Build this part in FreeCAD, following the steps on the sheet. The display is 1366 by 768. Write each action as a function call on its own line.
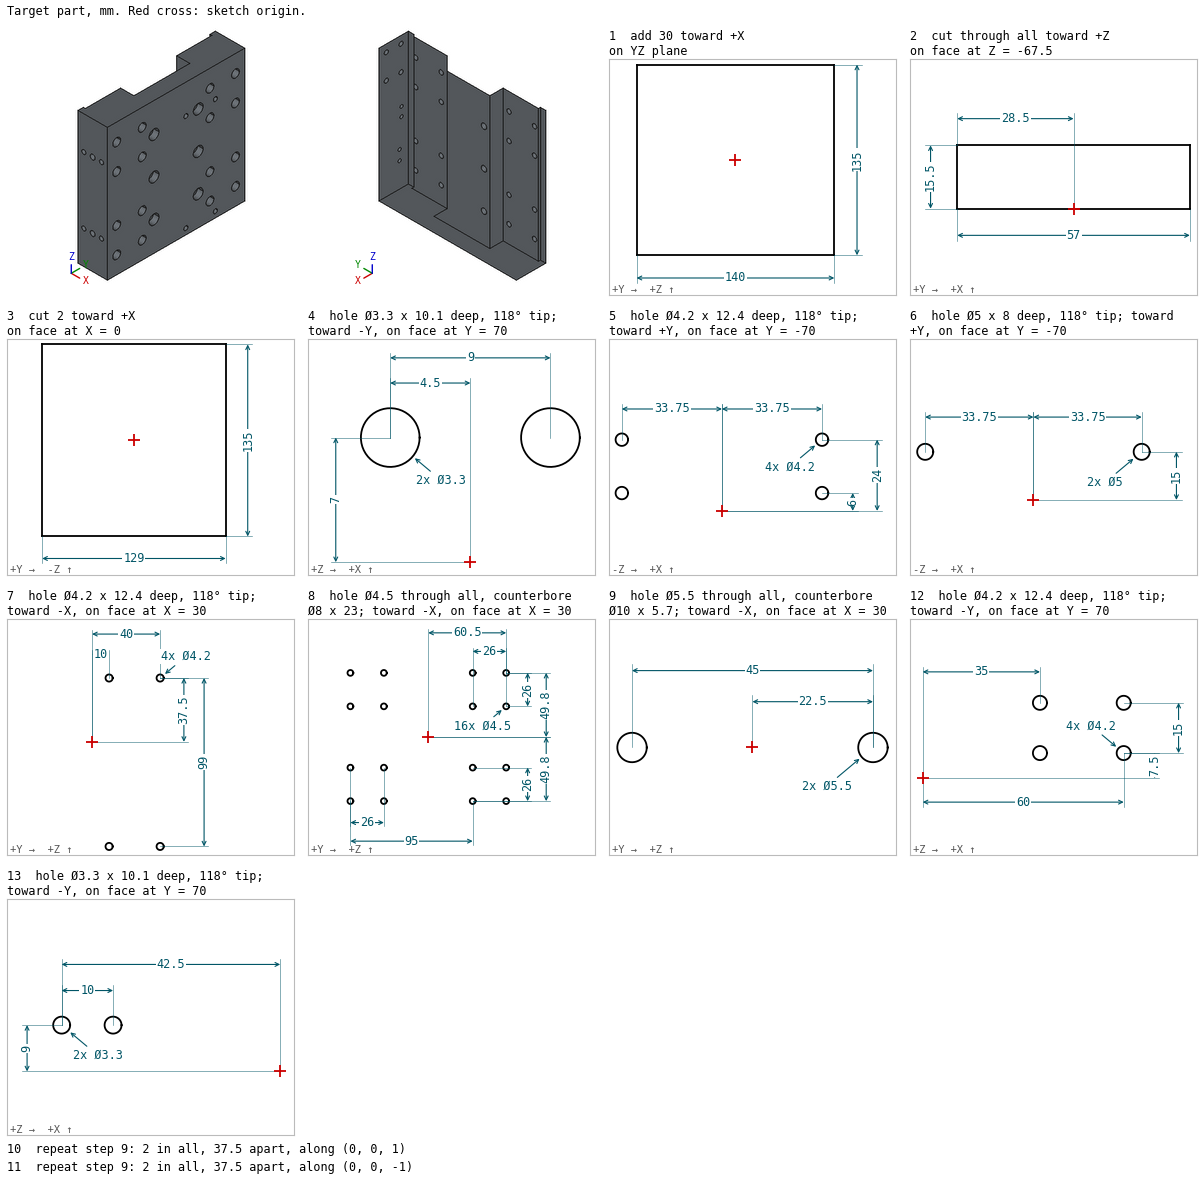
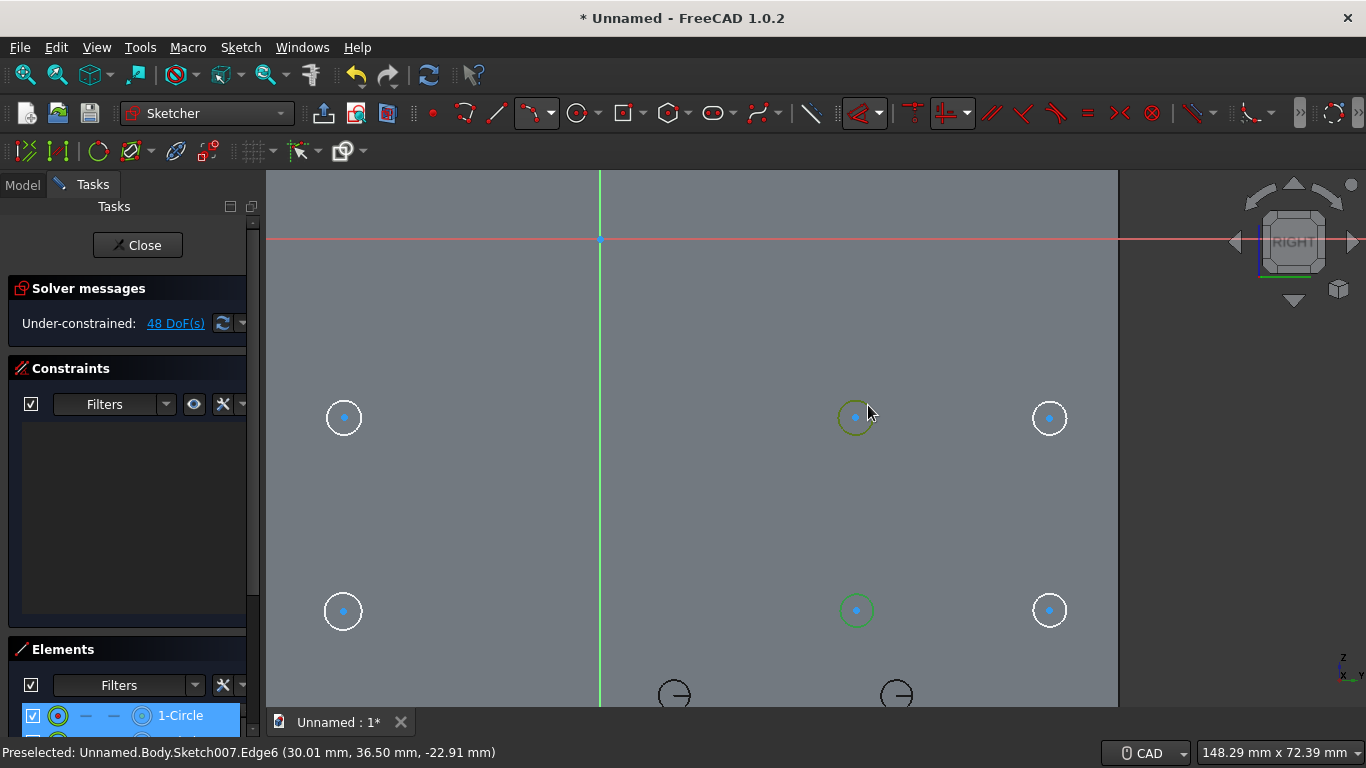
click(1062, 406)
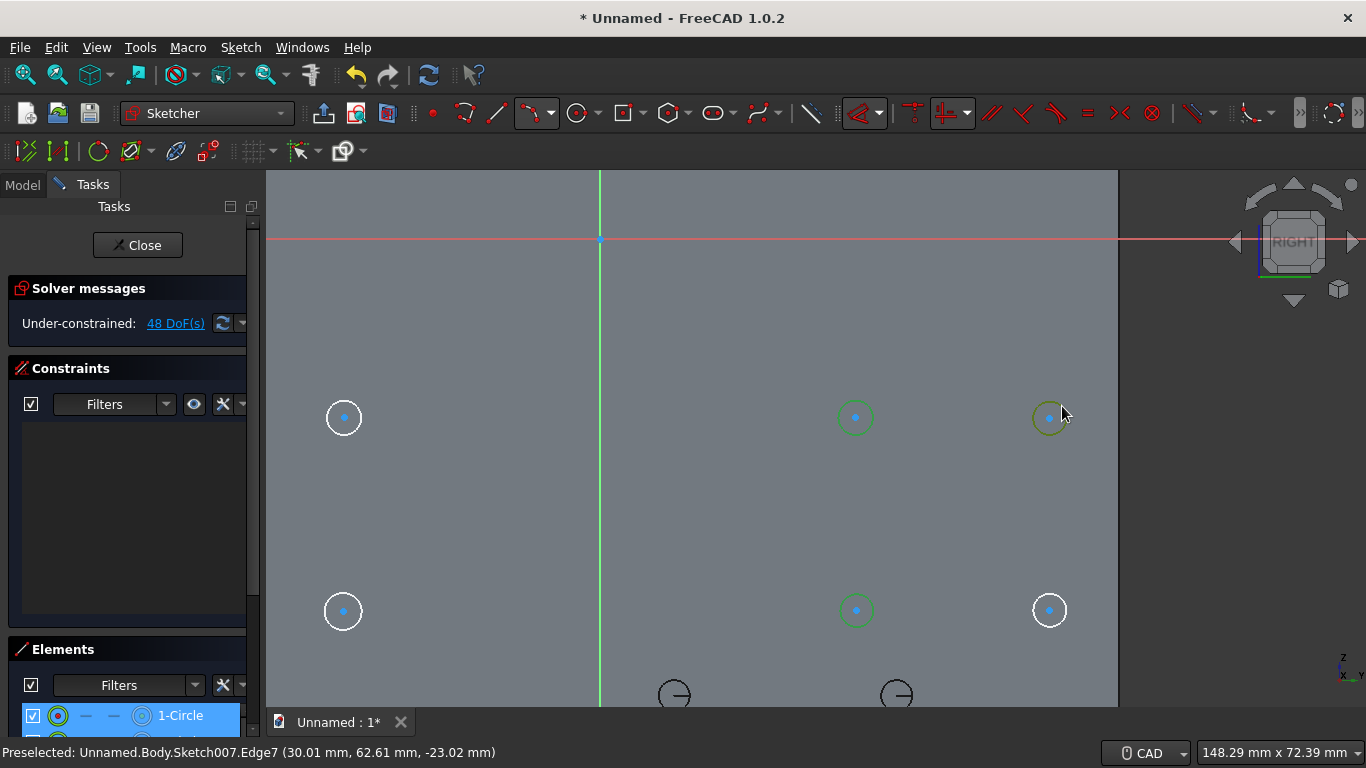
click(1061, 599)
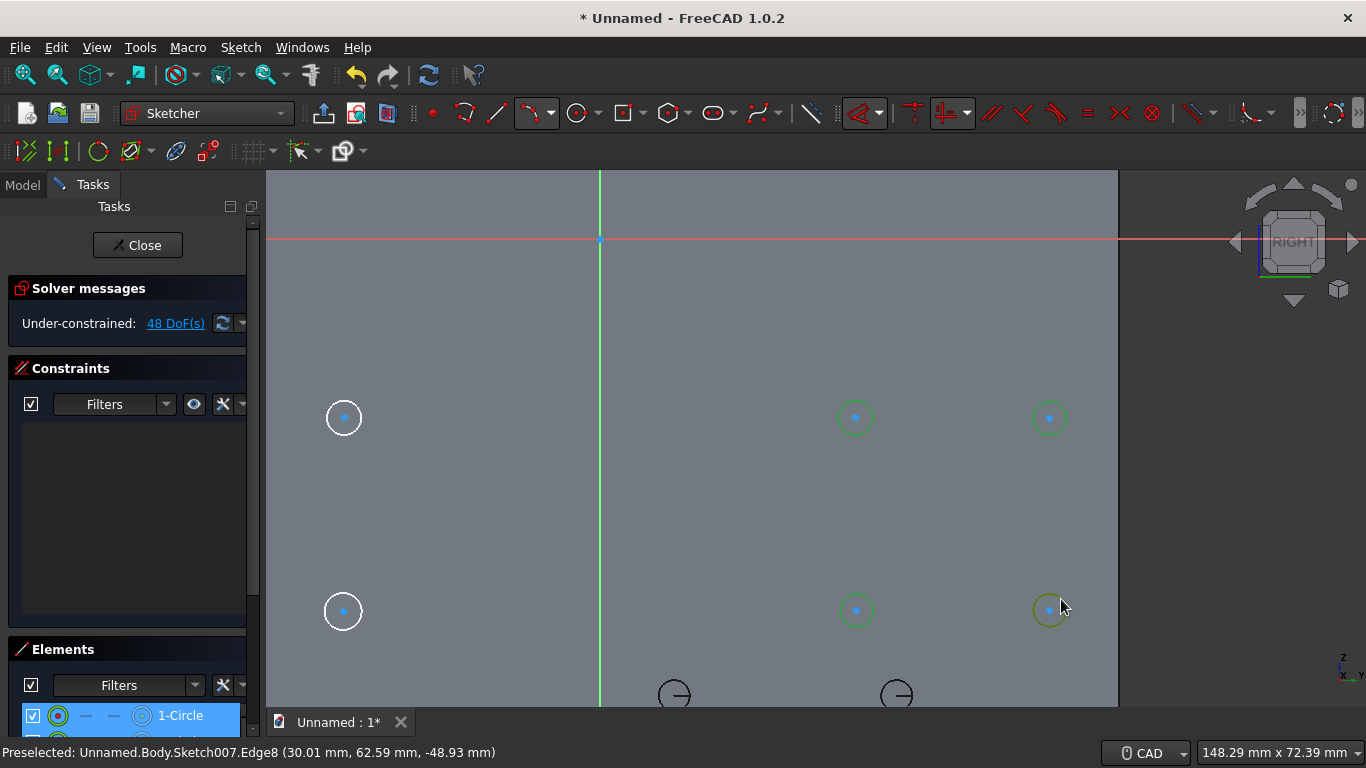
scroll(868, 601, down, 4)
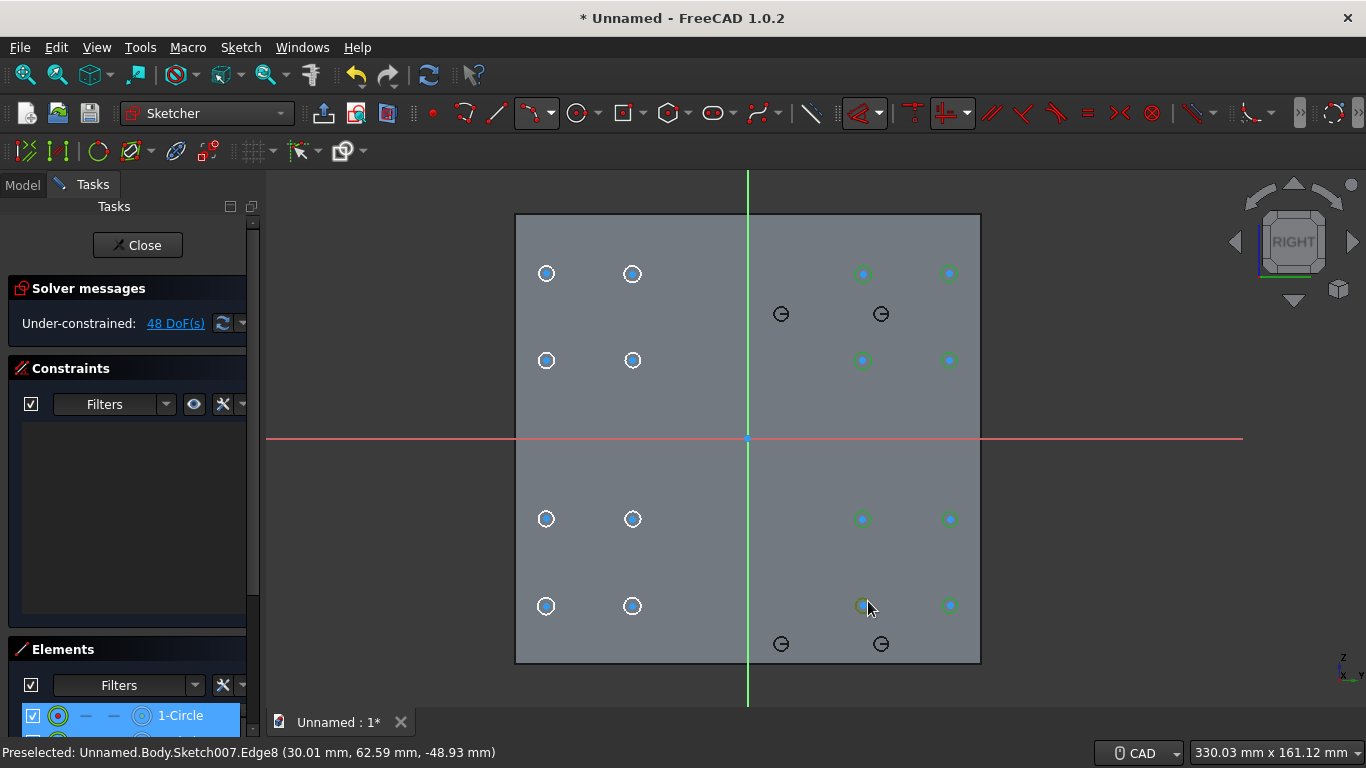
scroll(552, 600, up, 3)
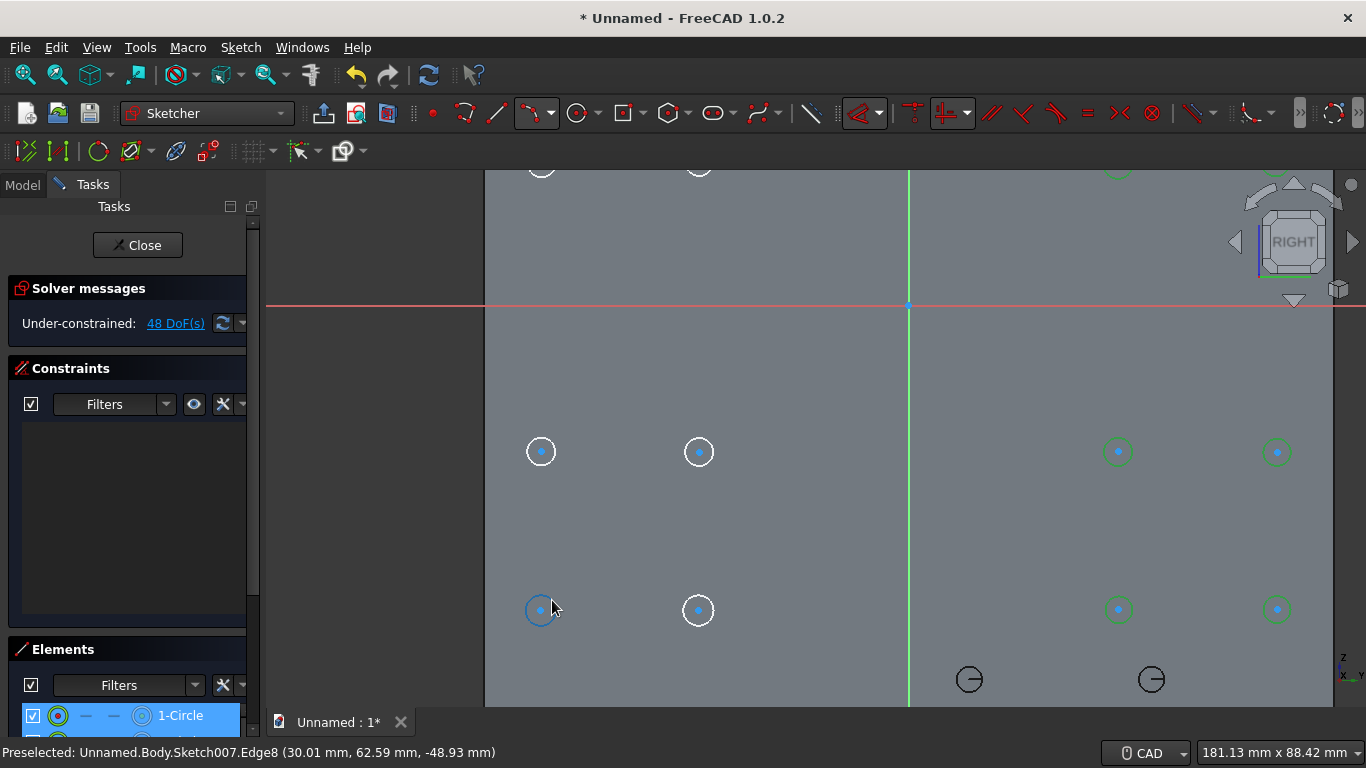
click(552, 600)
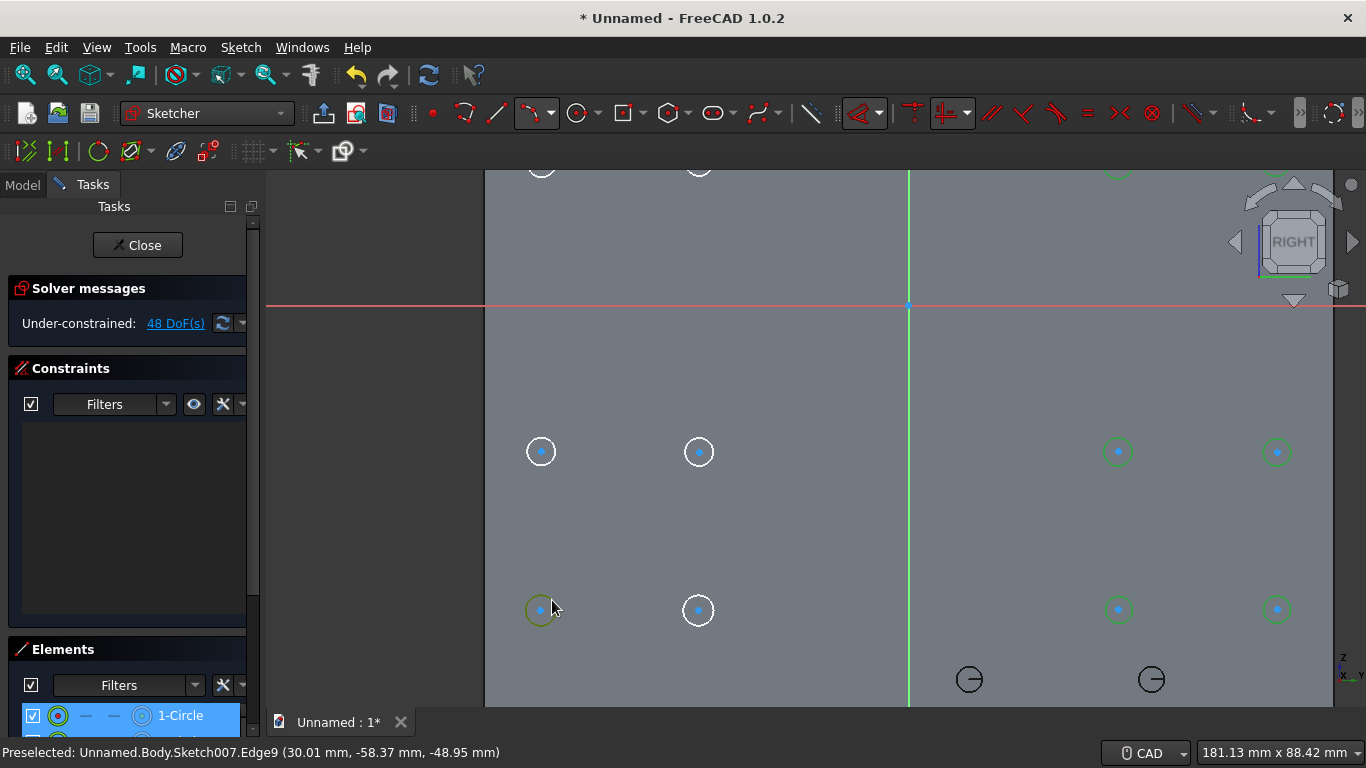
click(551, 442)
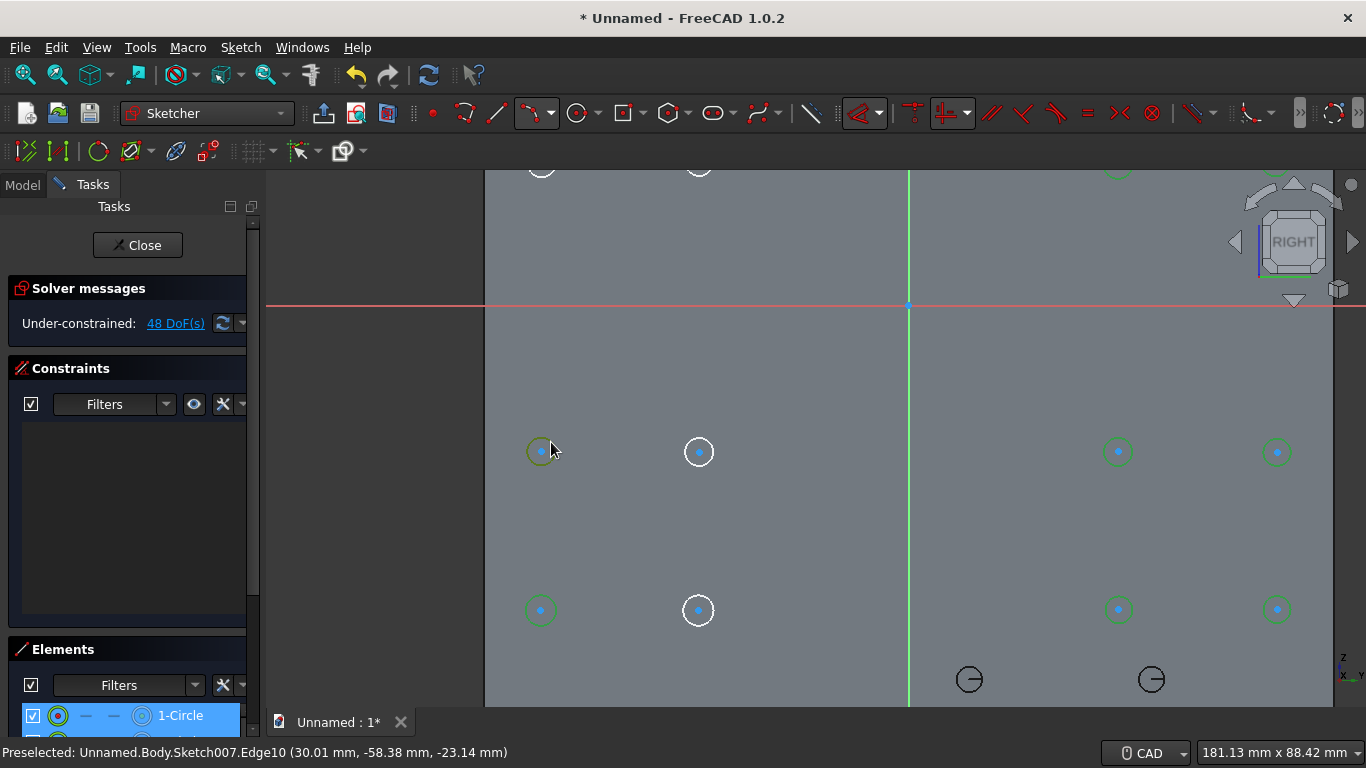
click(709, 442)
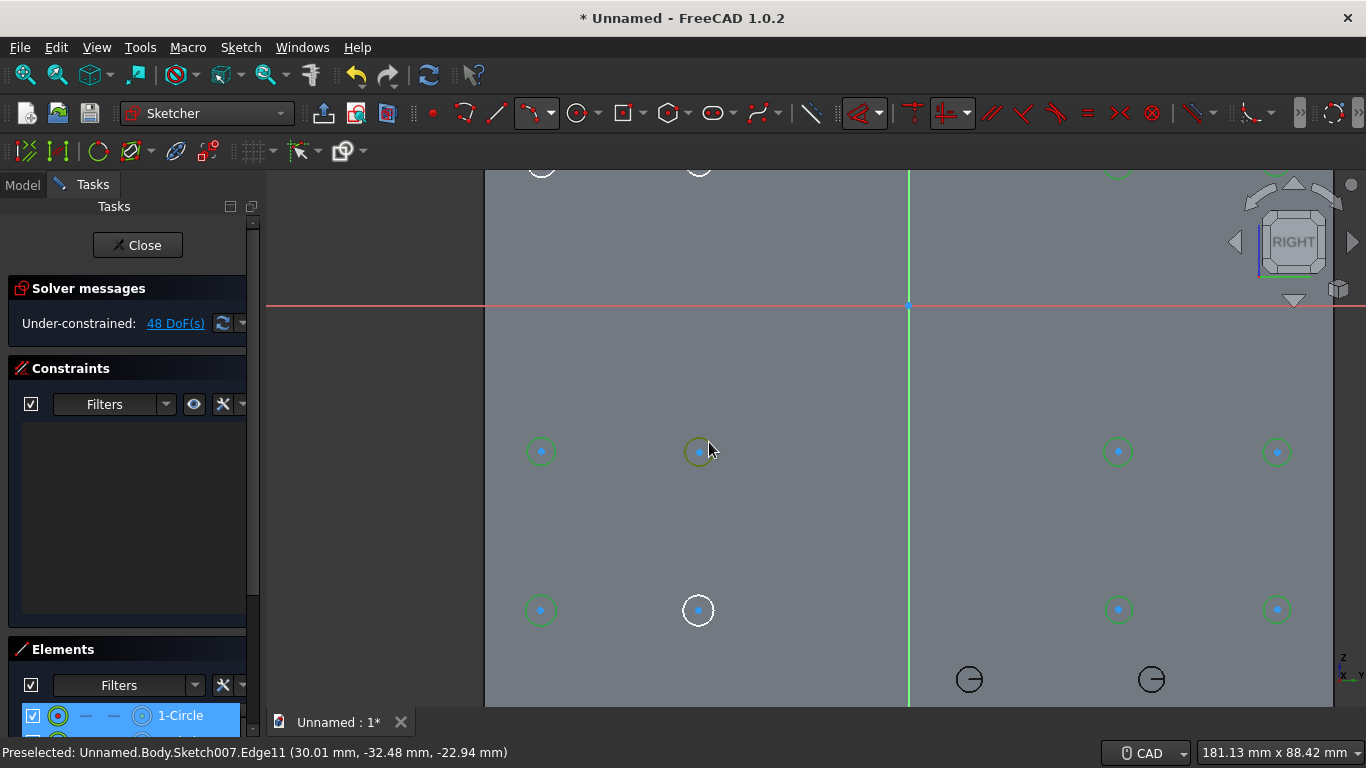
click(709, 600)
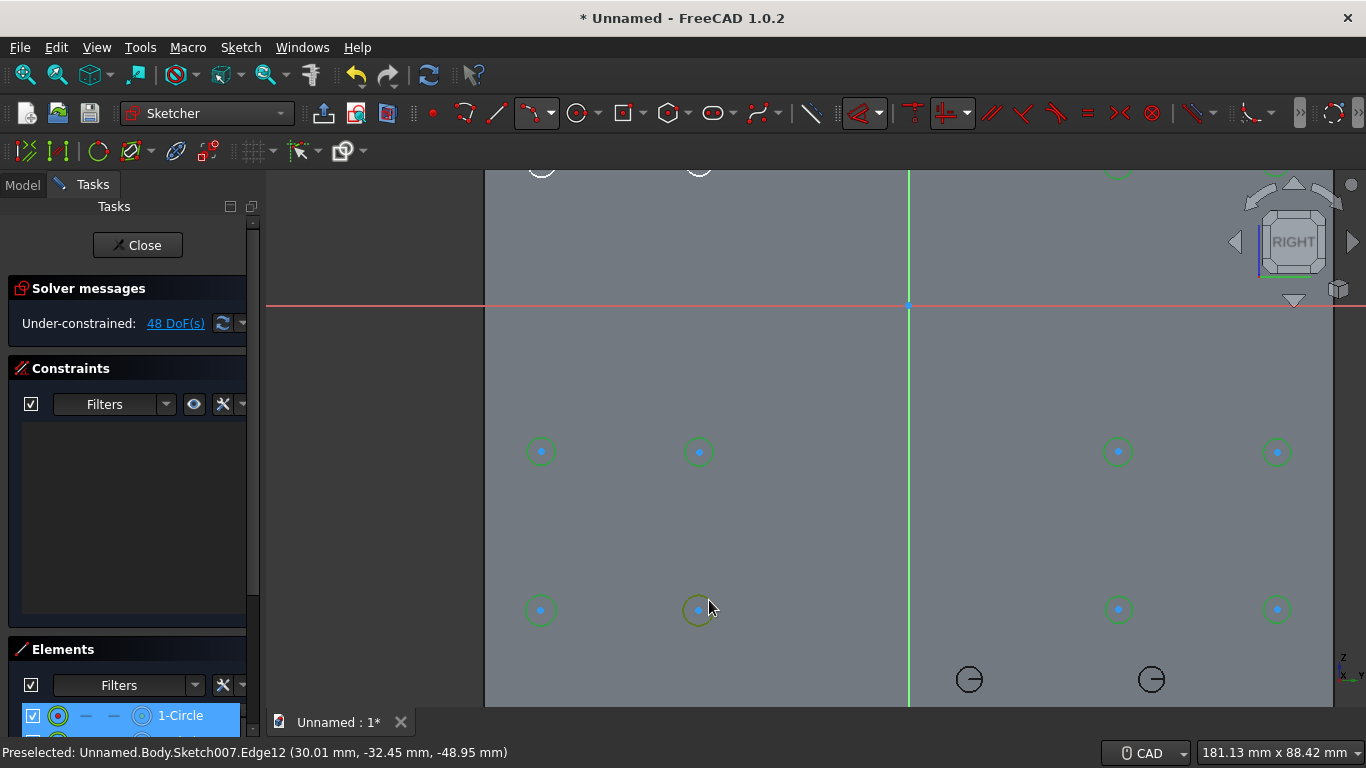
scroll(551, 600, down, 3)